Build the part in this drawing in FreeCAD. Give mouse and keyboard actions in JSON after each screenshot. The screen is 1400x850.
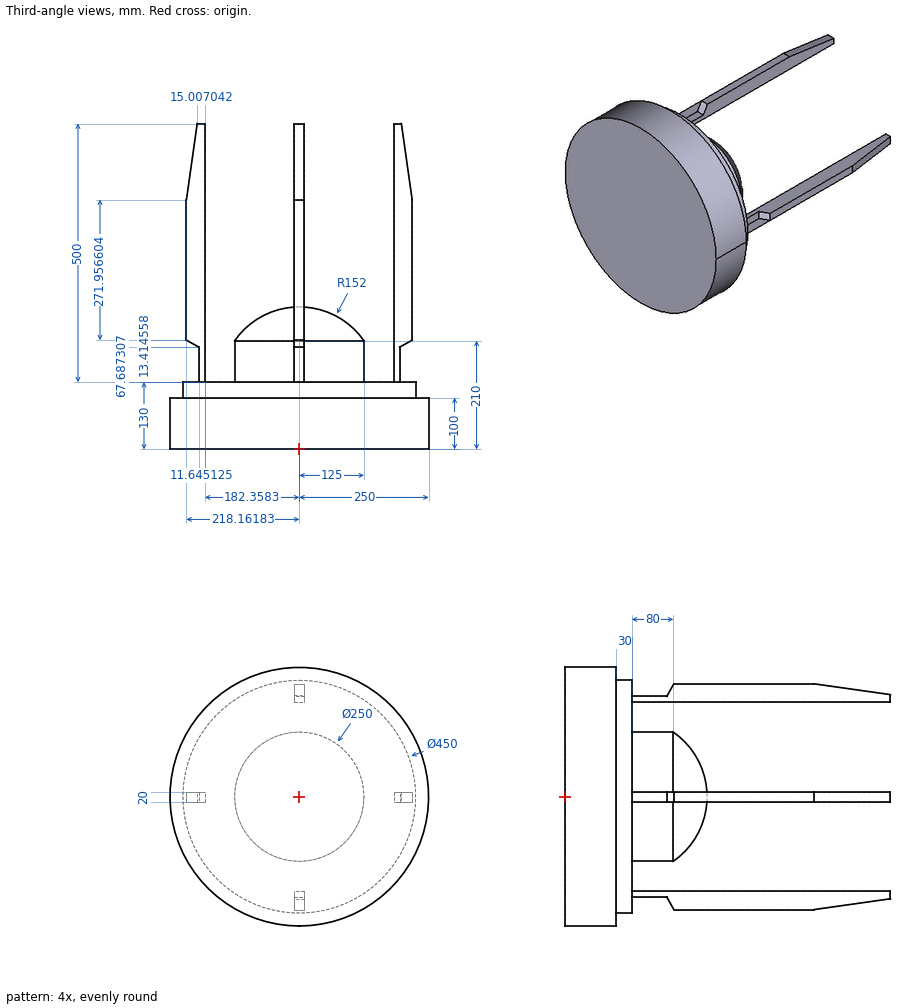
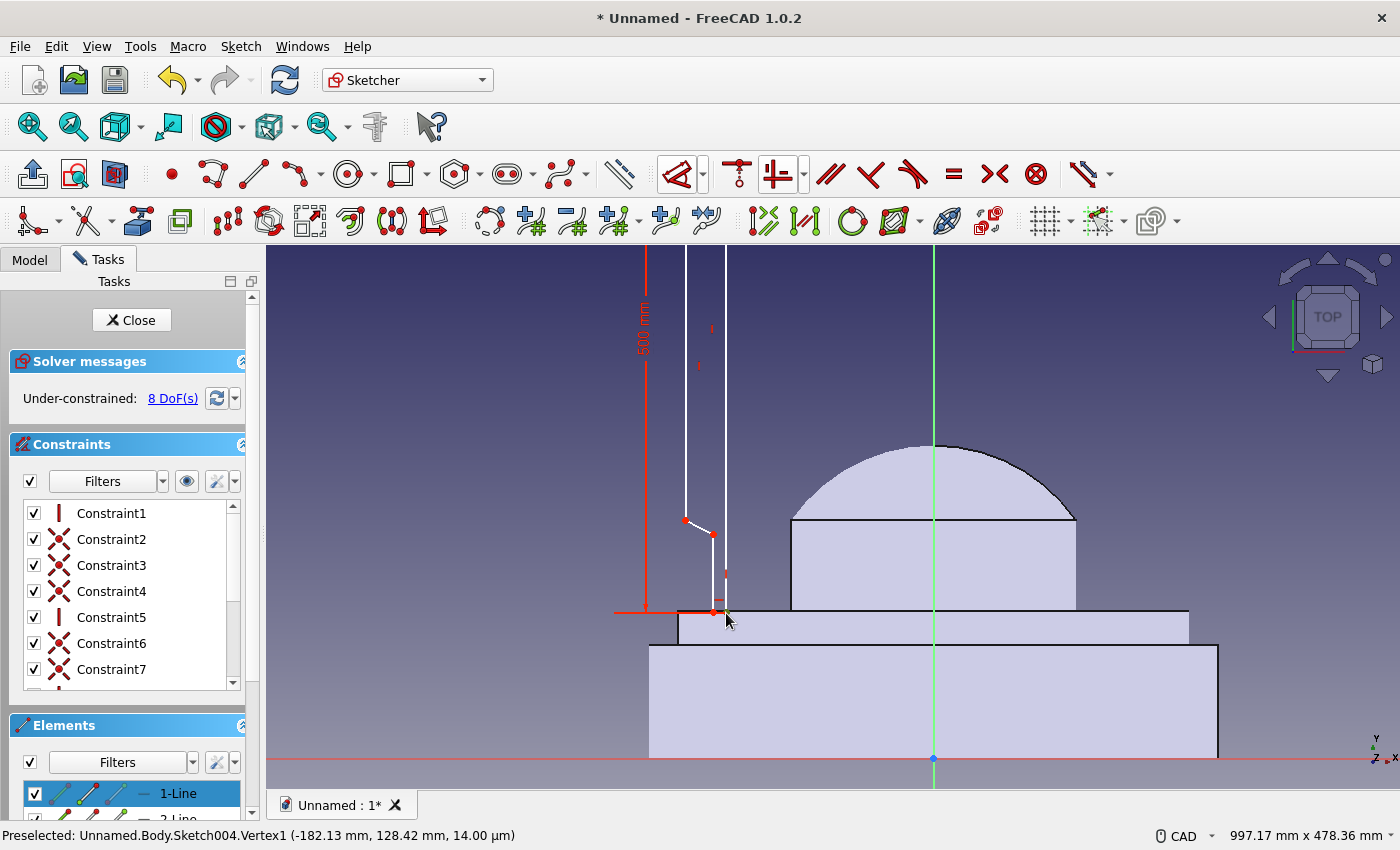
{"action": "left_click", "coordinate": [702, 174]}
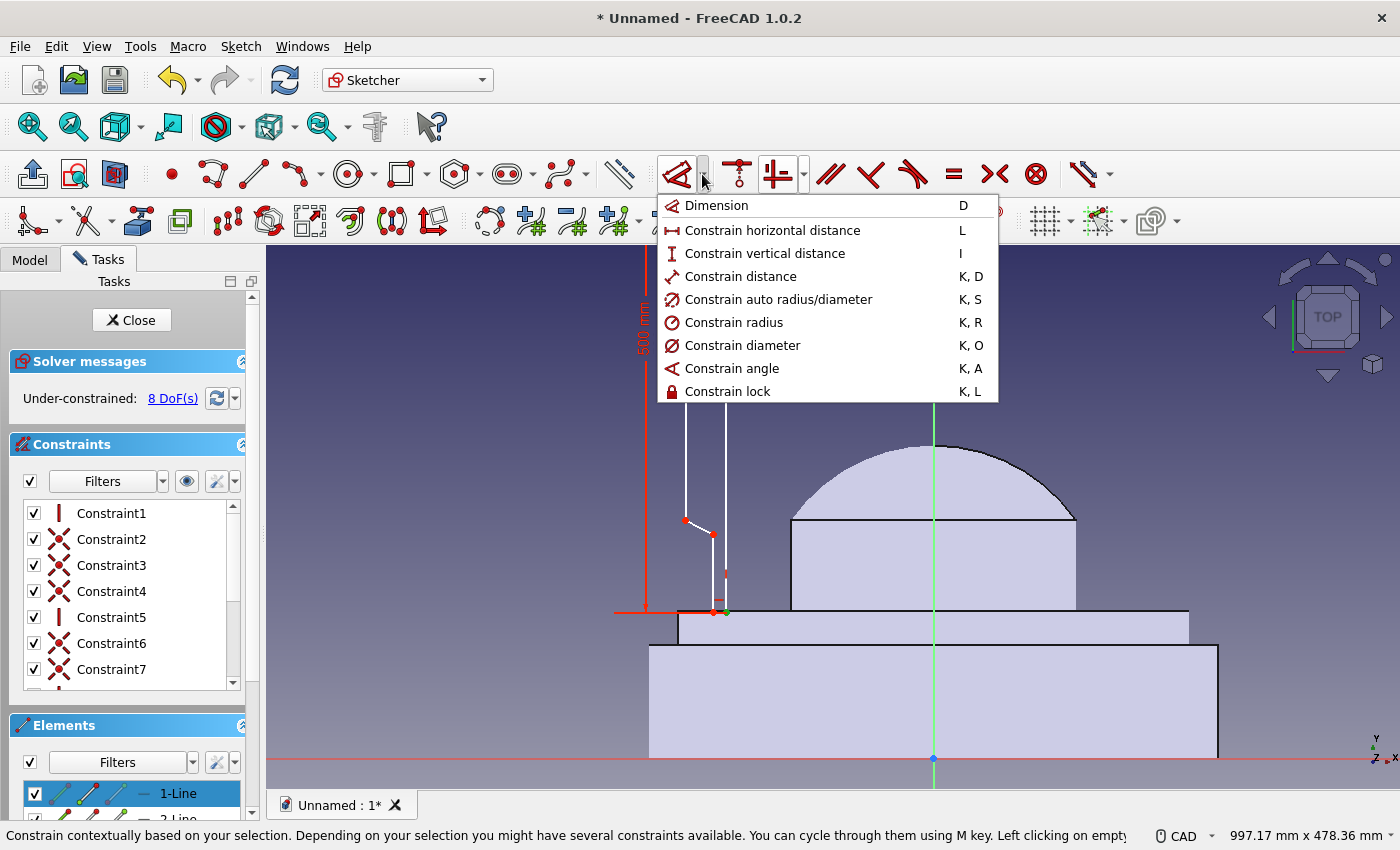
{"action": "left_click", "coordinate": [828, 254]}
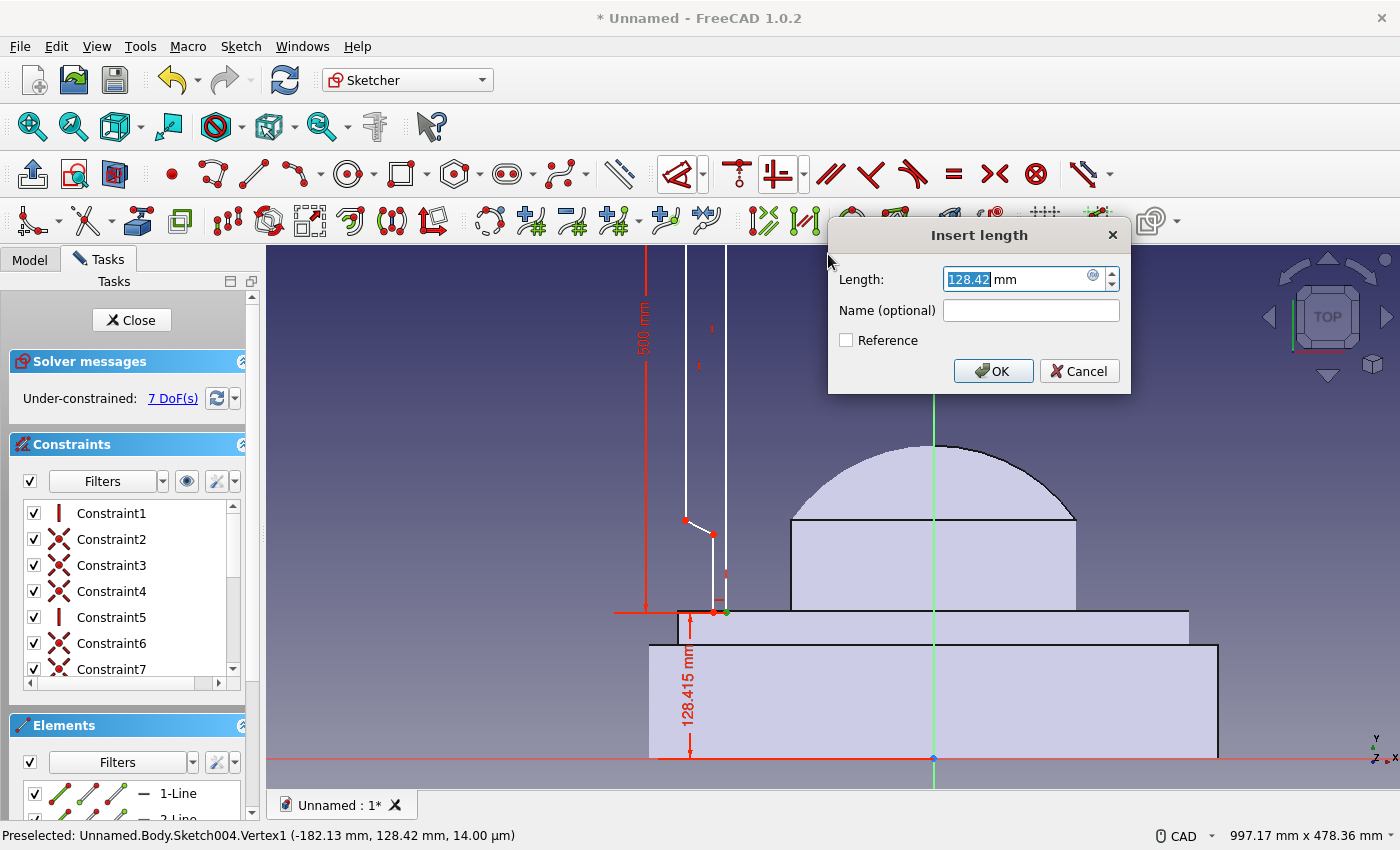
{"action": "type", "text": "130"}
{"action": "key", "text": "Return"}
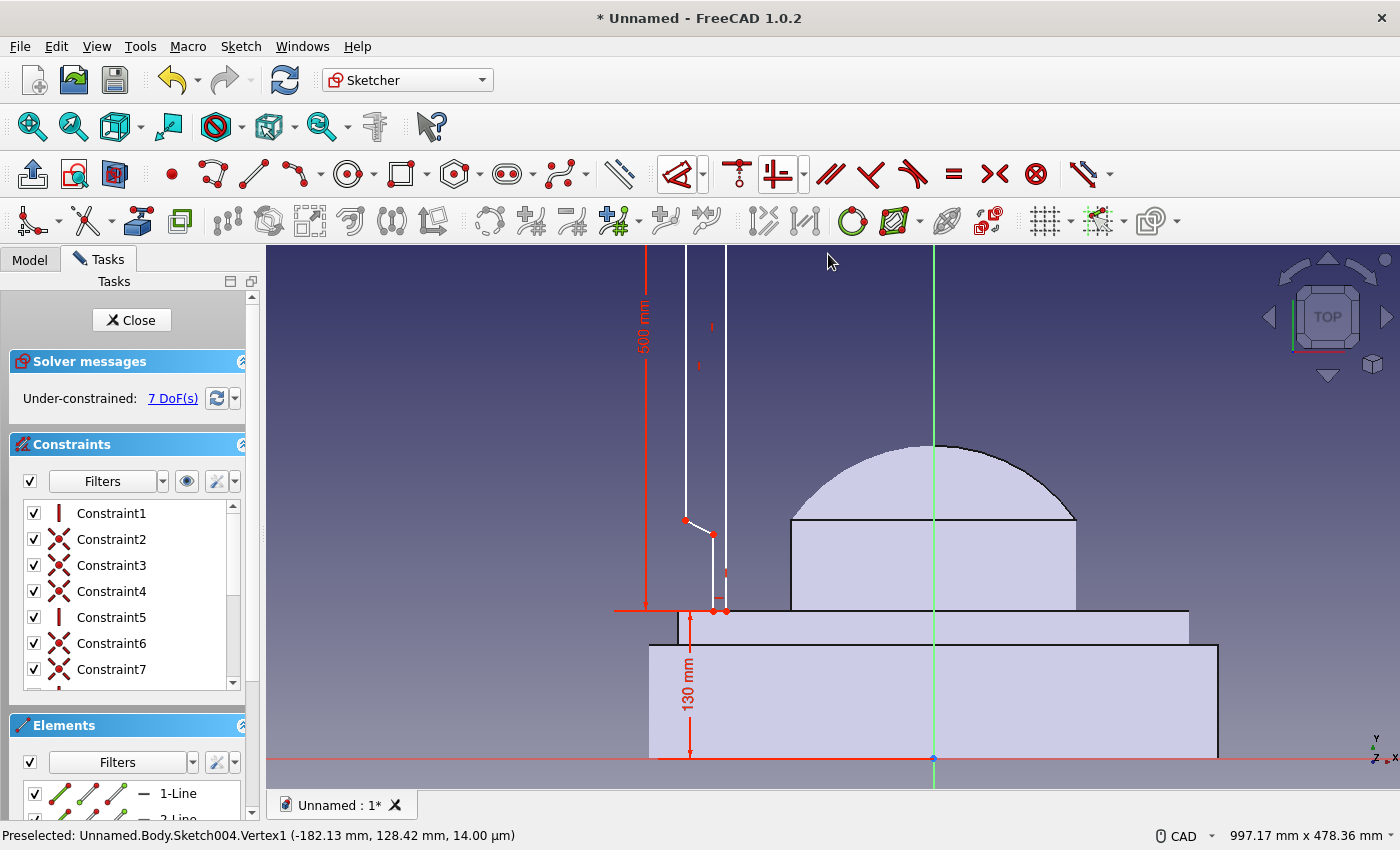
{"action": "scroll", "coordinate": [728, 612], "scroll_direction": "down", "scroll_amount": 4}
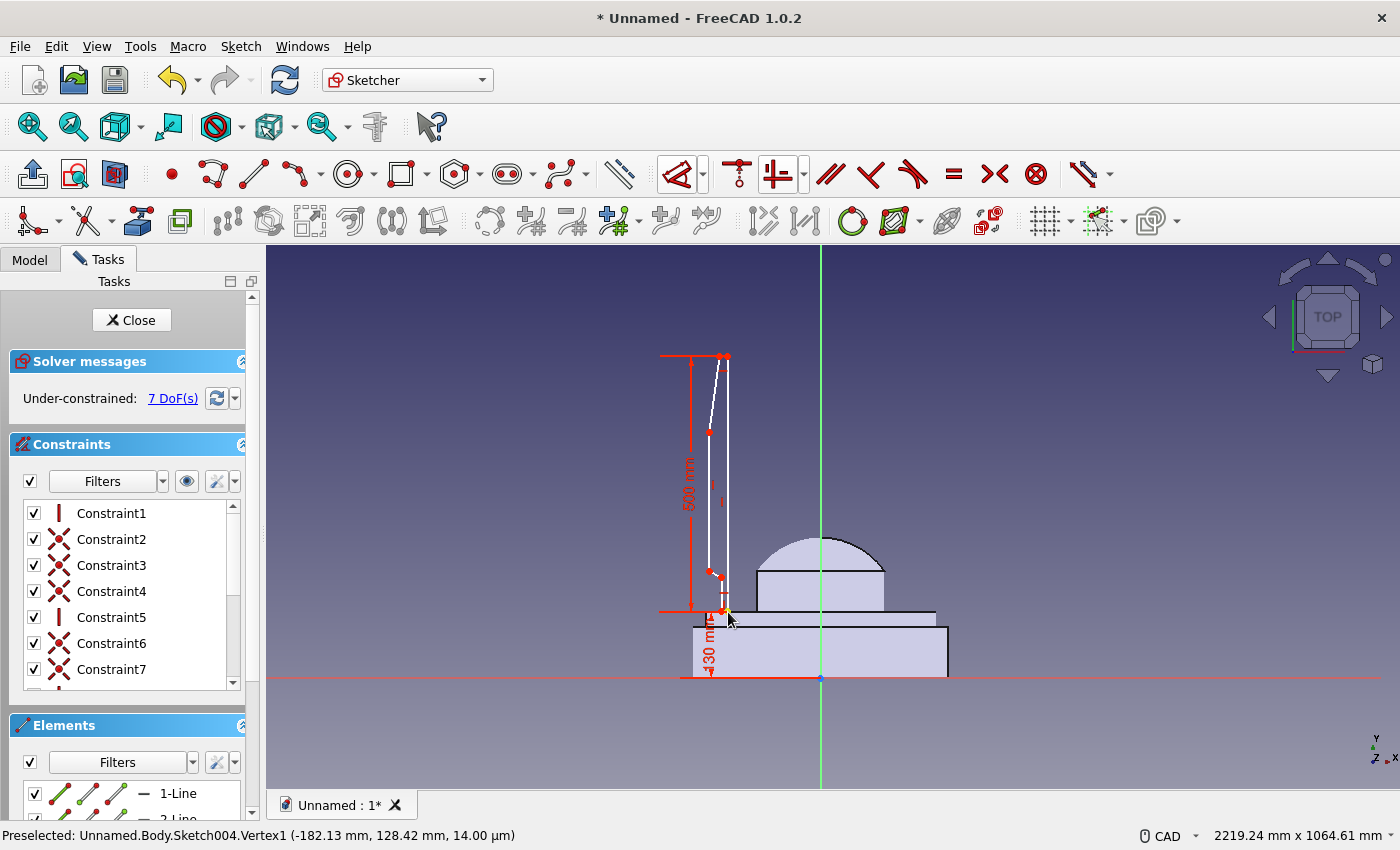
{"action": "scroll", "coordinate": [724, 356], "scroll_direction": "up", "scroll_amount": 9}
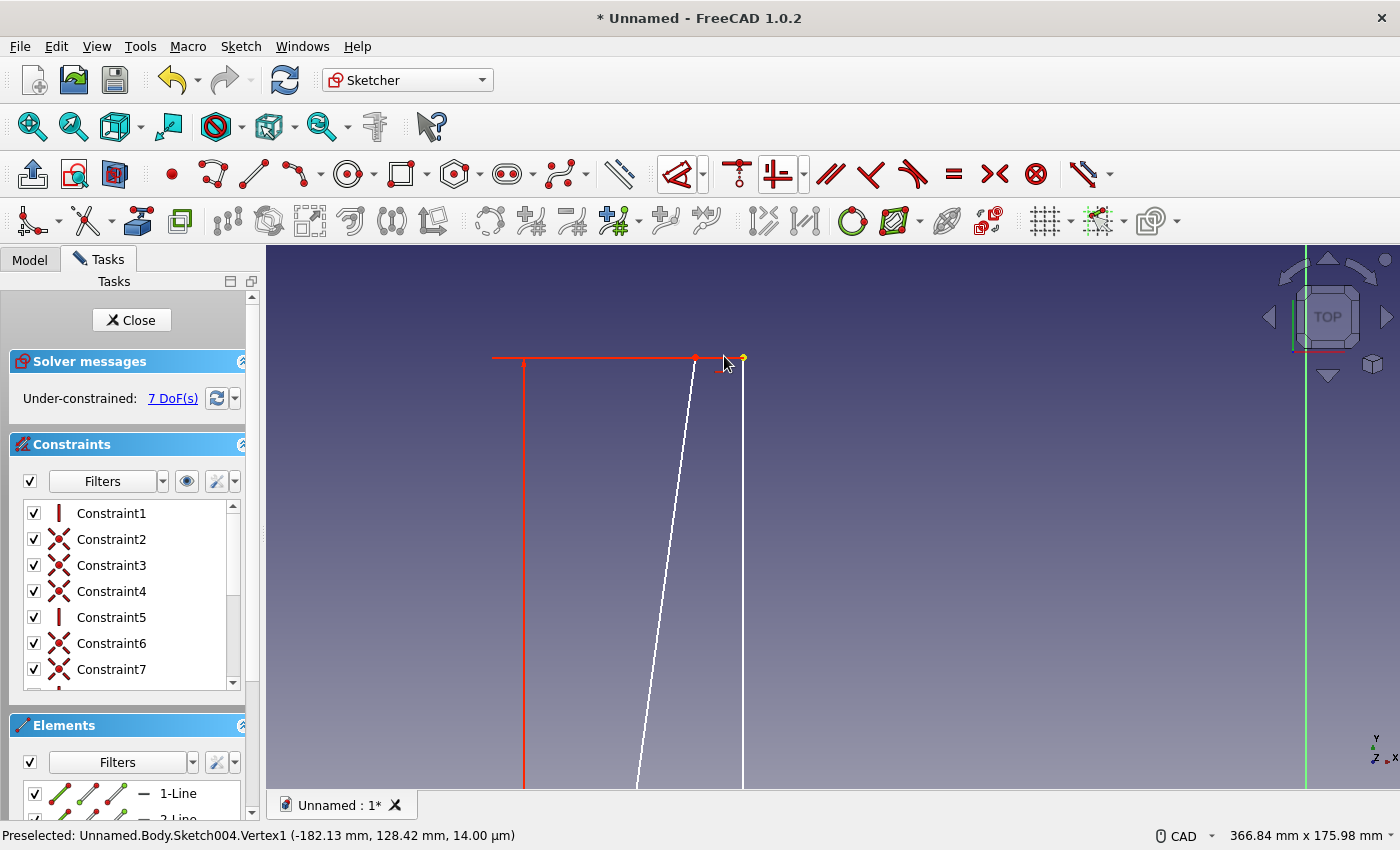
{"action": "left_click", "coordinate": [719, 358]}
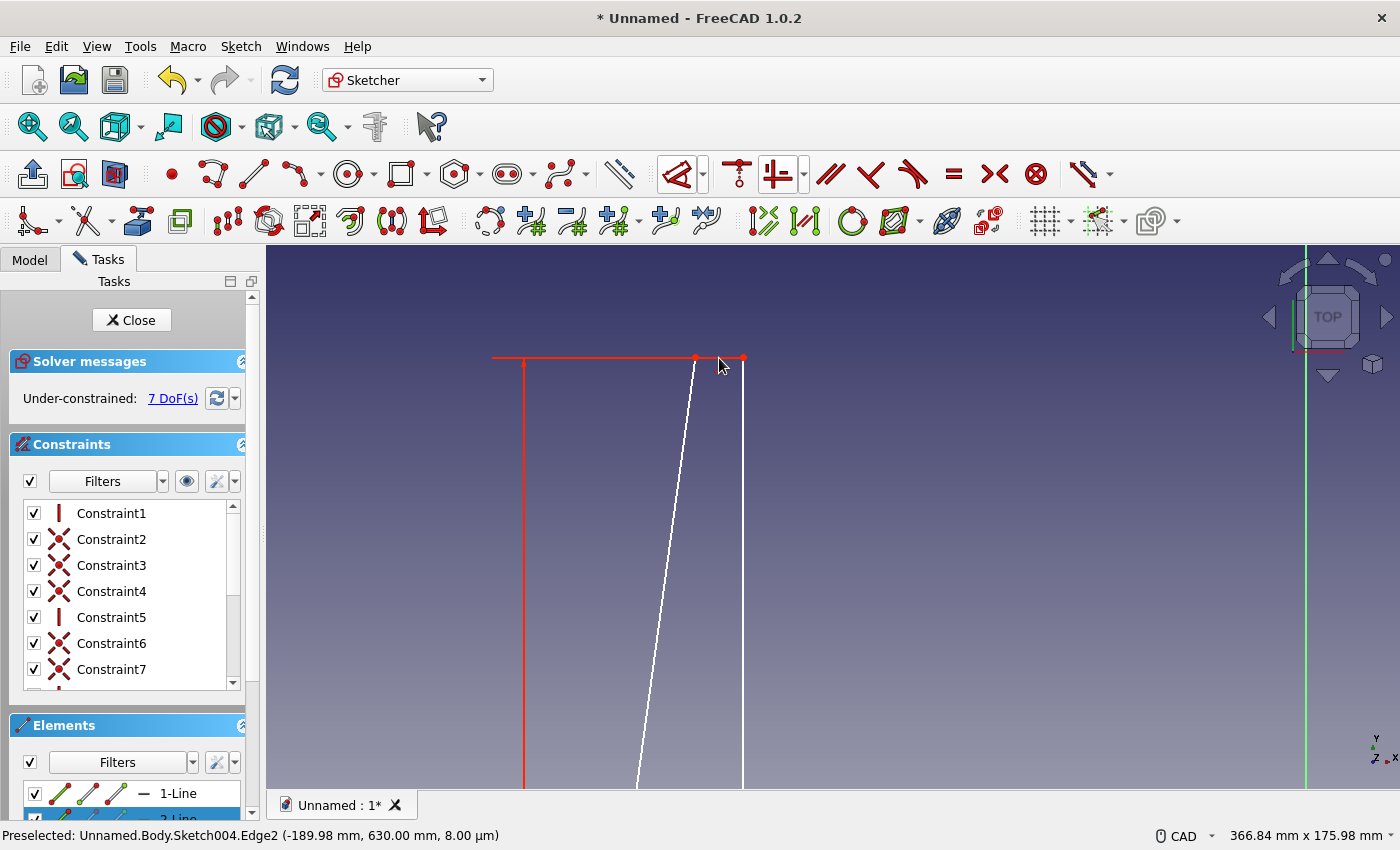
{"action": "key", "text": "l"}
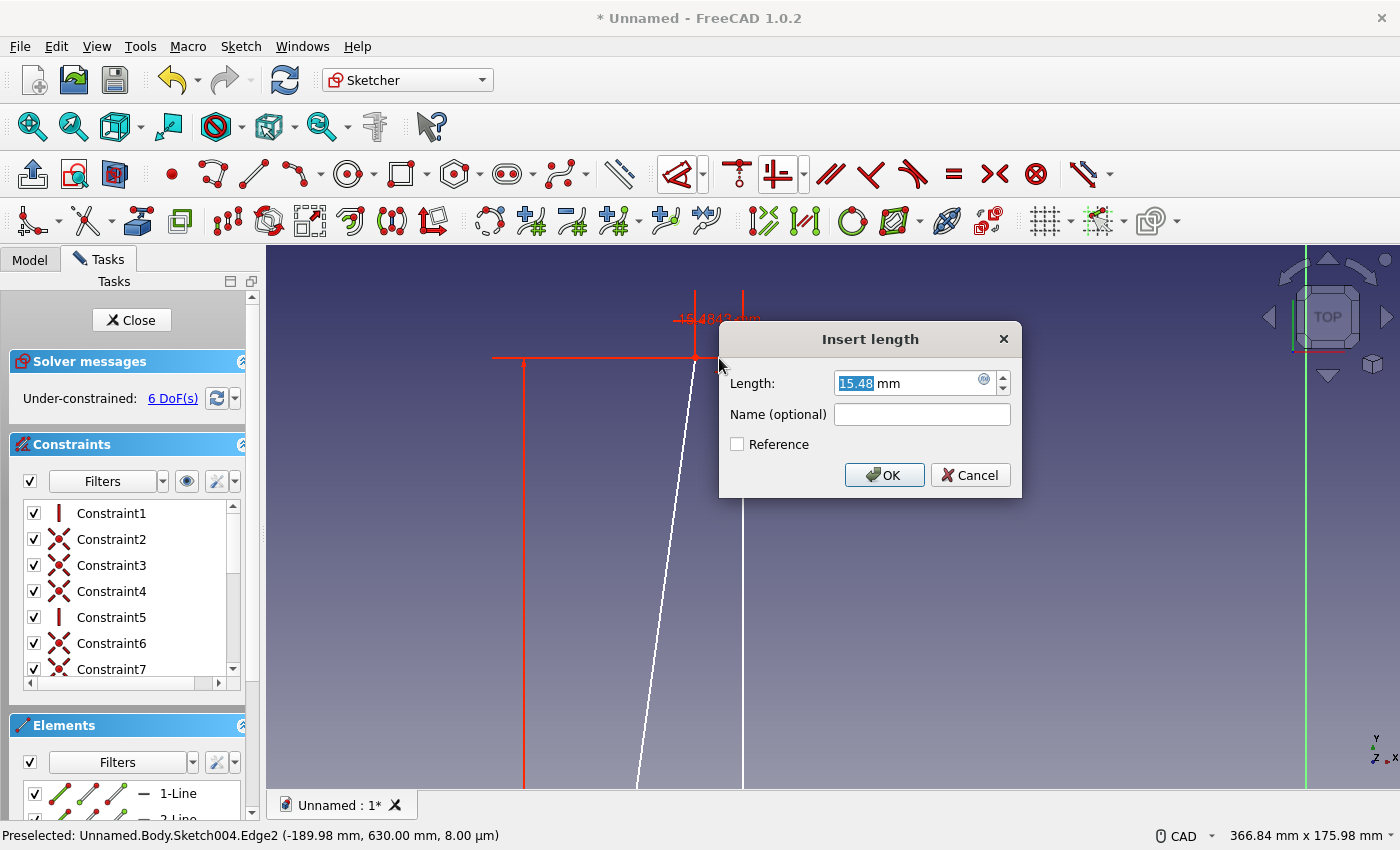
{"action": "type", "text": "15.007042"}
{"action": "key", "text": "Return"}